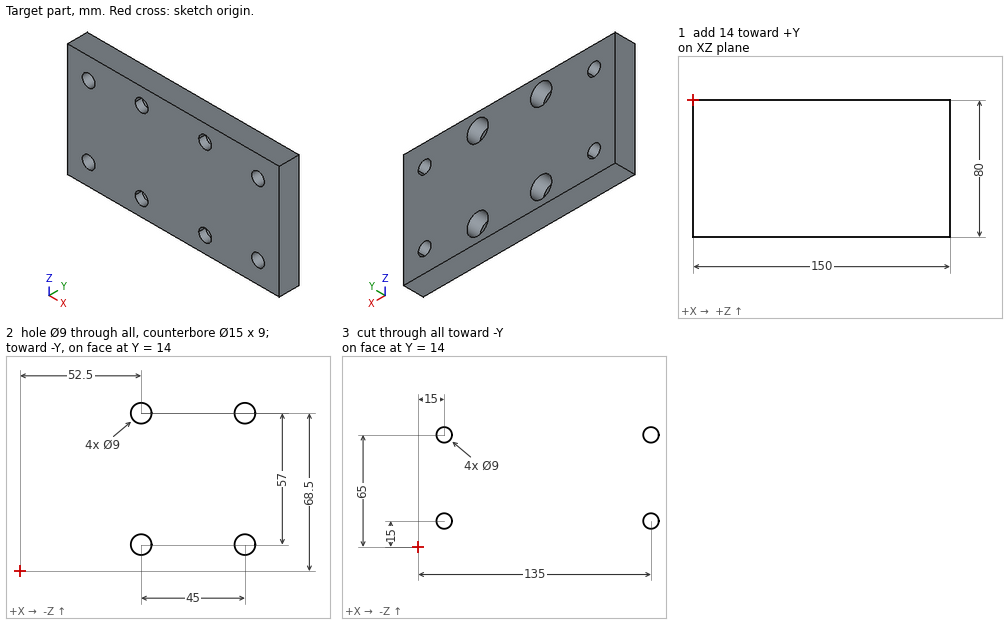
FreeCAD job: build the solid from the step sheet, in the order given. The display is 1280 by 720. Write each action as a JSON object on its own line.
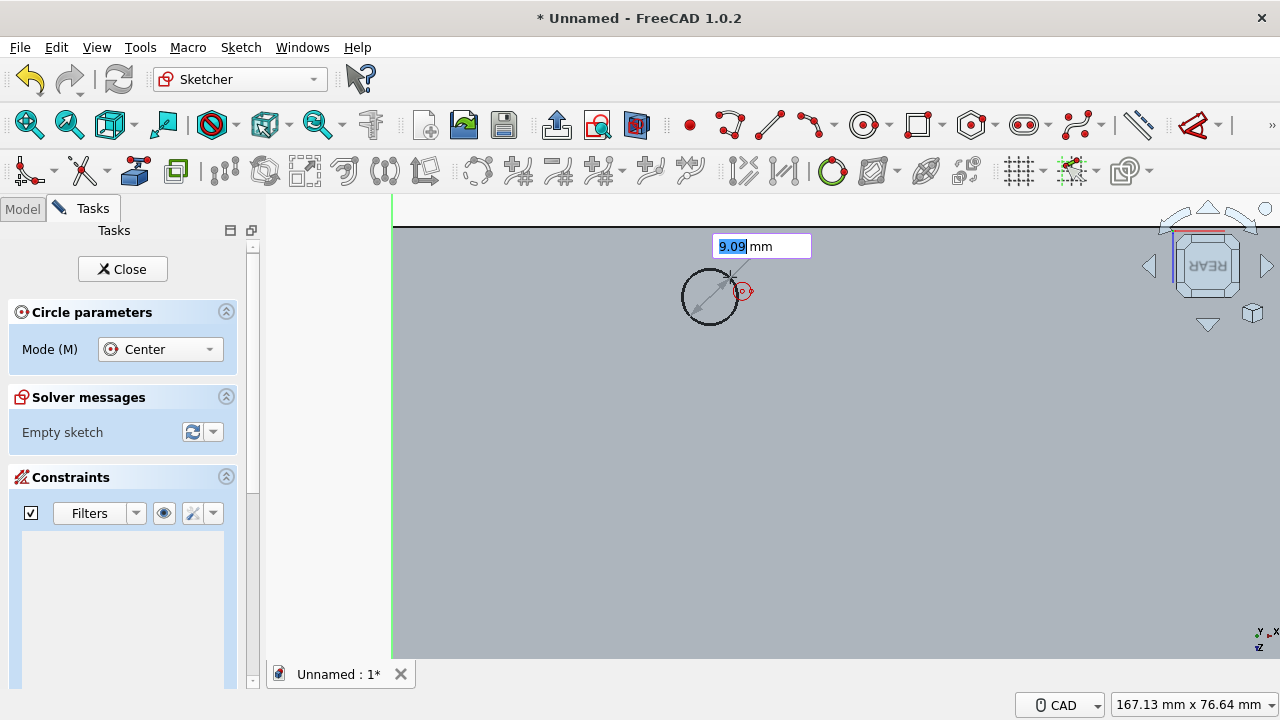
{"action": "type", "text": "9"}
{"action": "key", "text": "Return"}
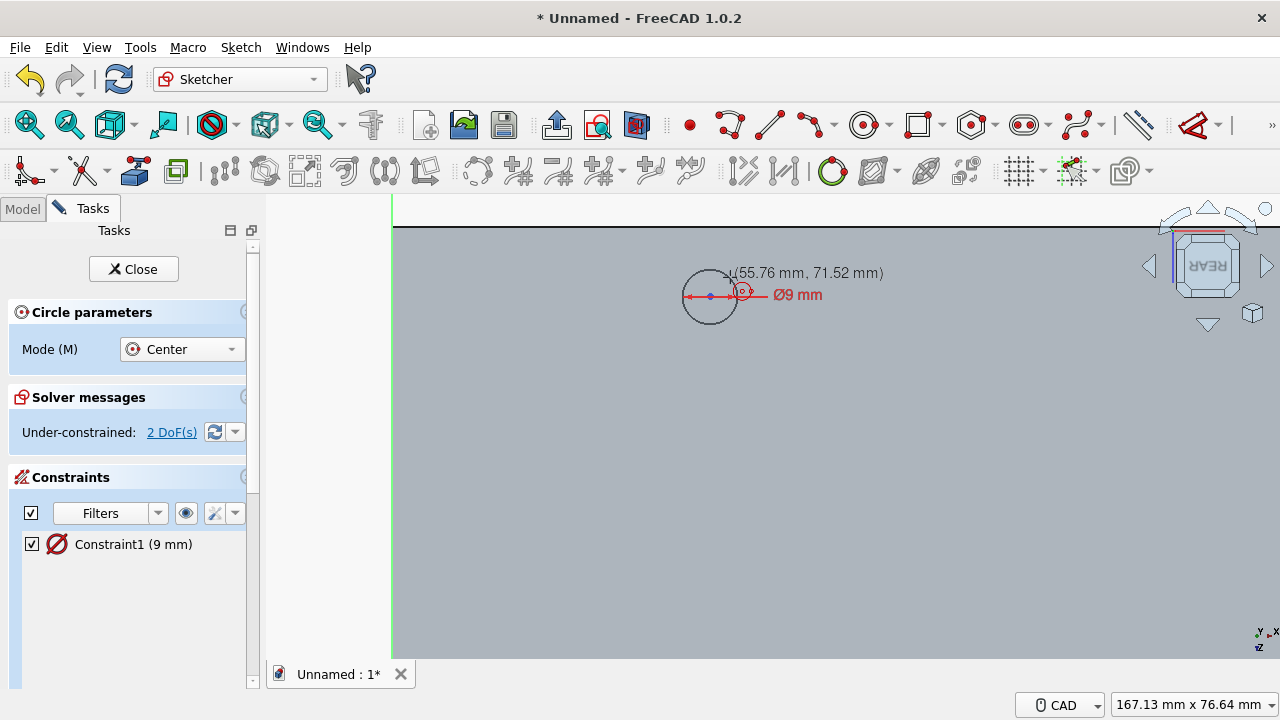
{"action": "scroll", "coordinate": [711, 296], "scroll_direction": "down", "scroll_amount": 2}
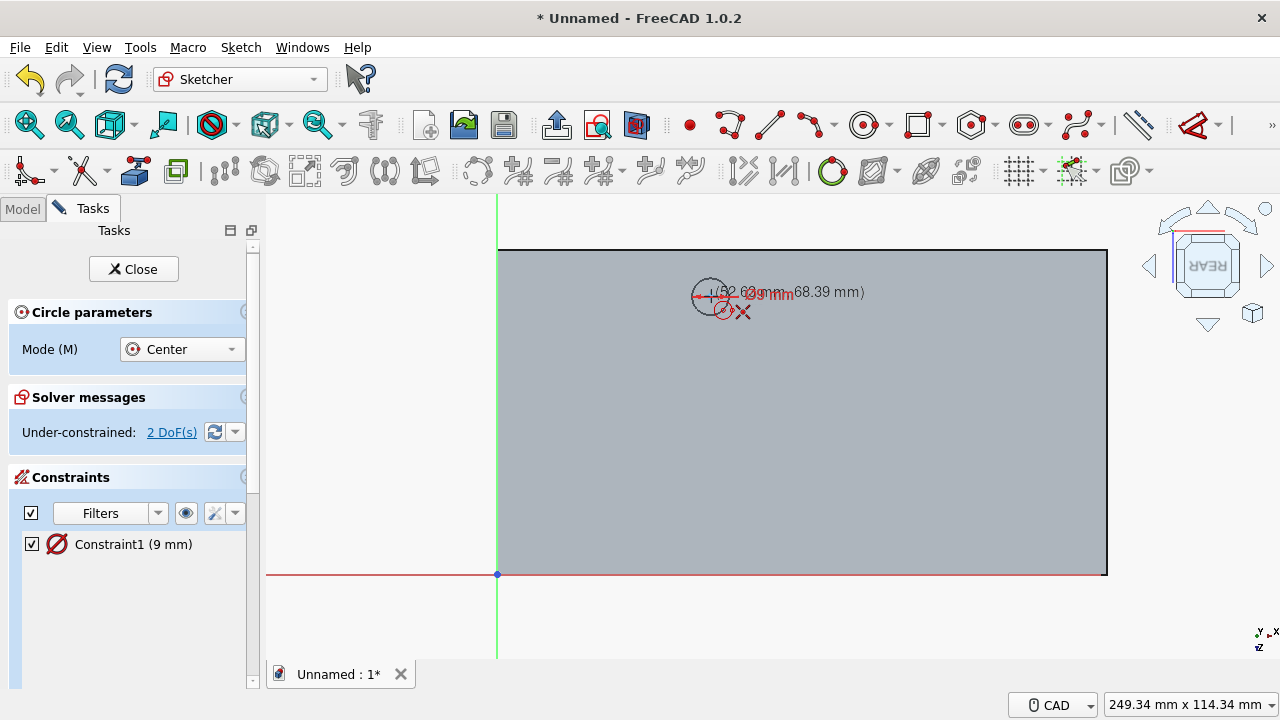
{"action": "scroll", "coordinate": [711, 528], "scroll_direction": "up", "scroll_amount": 2}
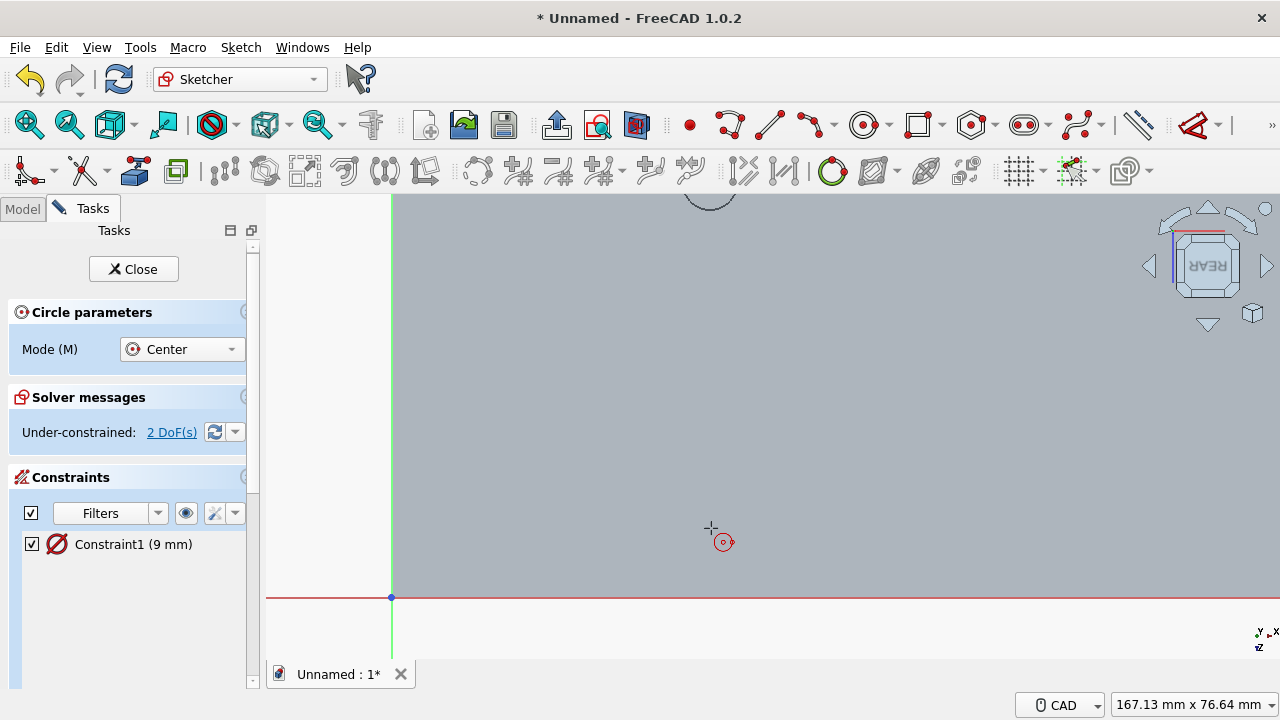
{"action": "left_click", "coordinate": [710, 528]}
{"action": "mouse_move", "coordinate": [730, 509]}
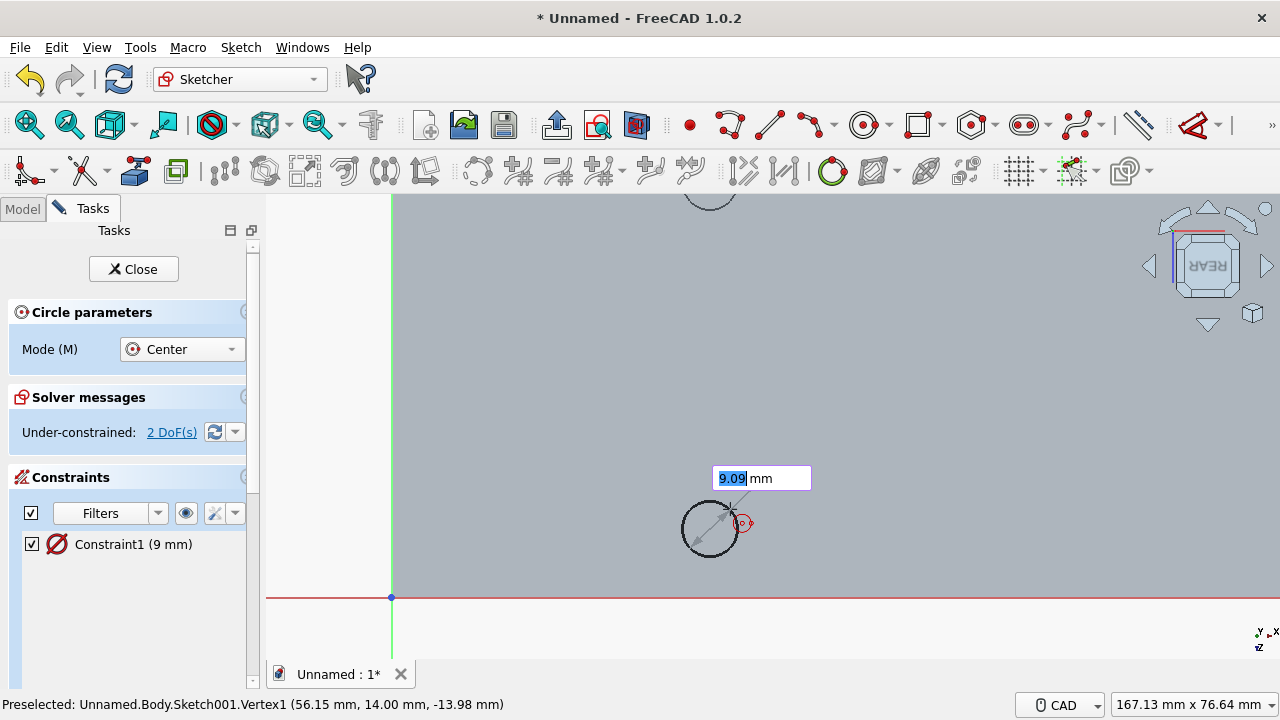
{"action": "type", "text": "9"}
{"action": "key", "text": "Return"}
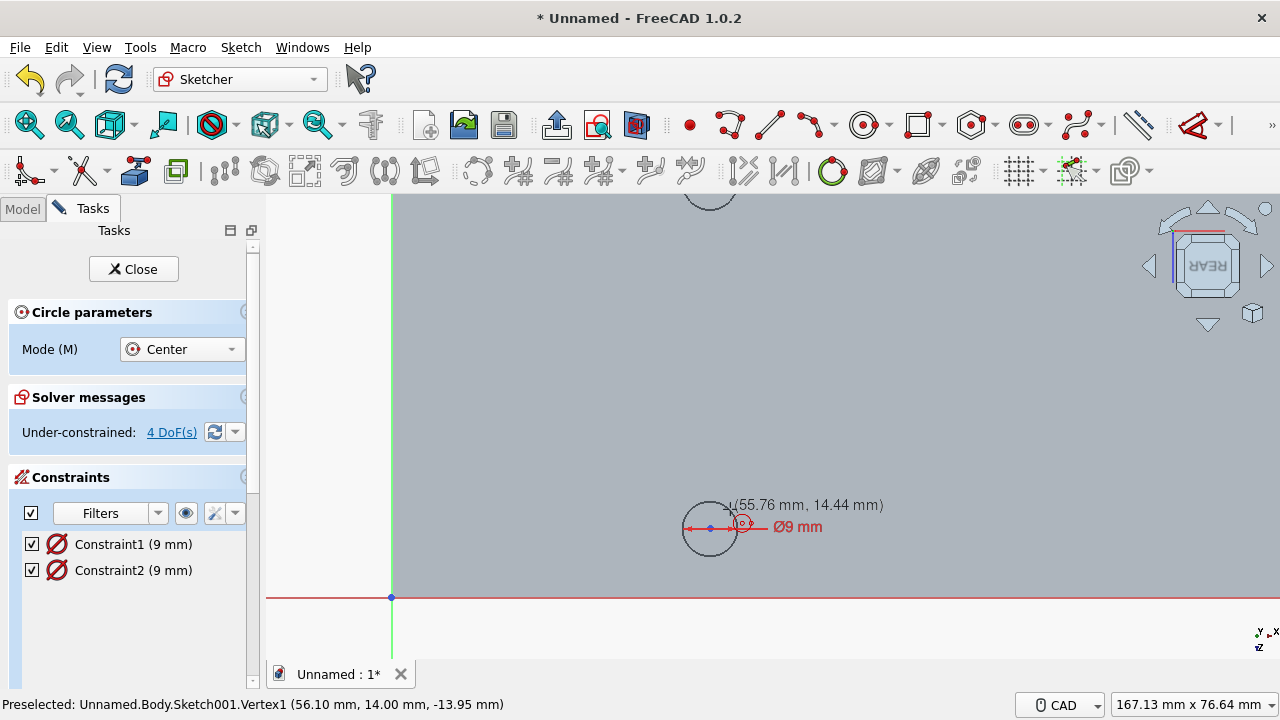
{"action": "left_click", "coordinate": [983, 528]}
{"action": "mouse_move", "coordinate": [1003, 509]}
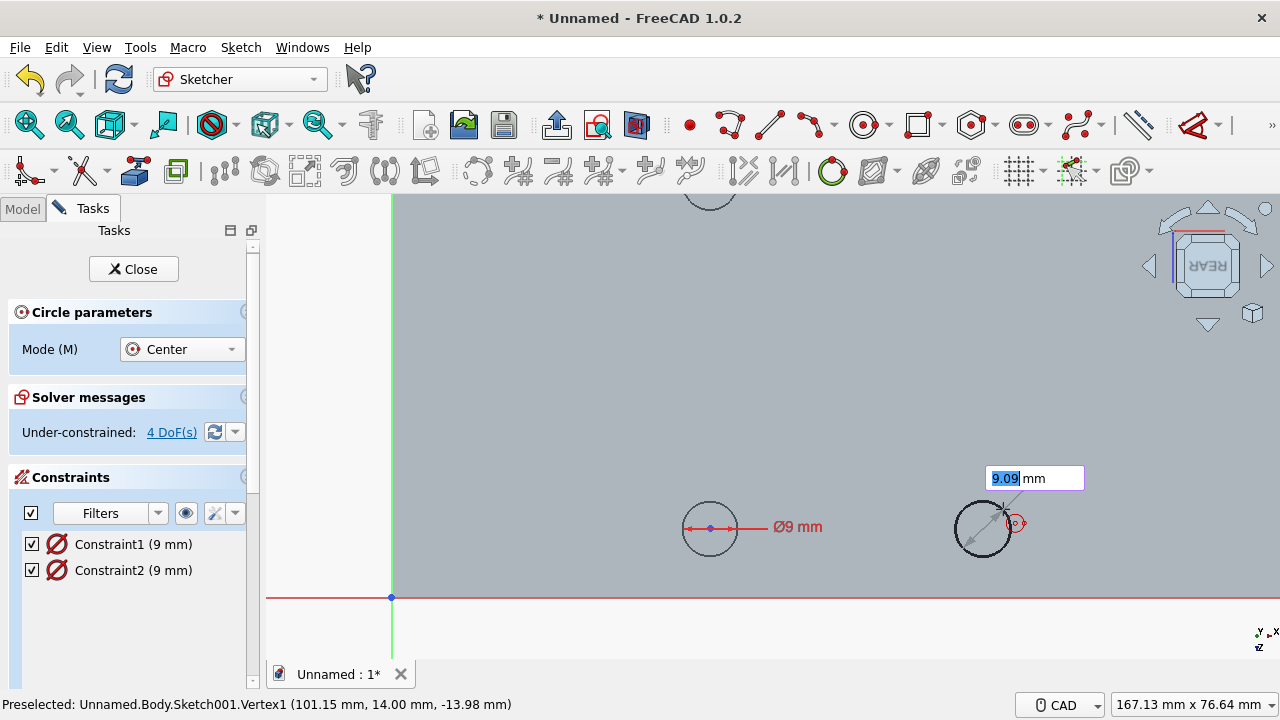
{"action": "type", "text": "9"}
{"action": "key", "text": "Return"}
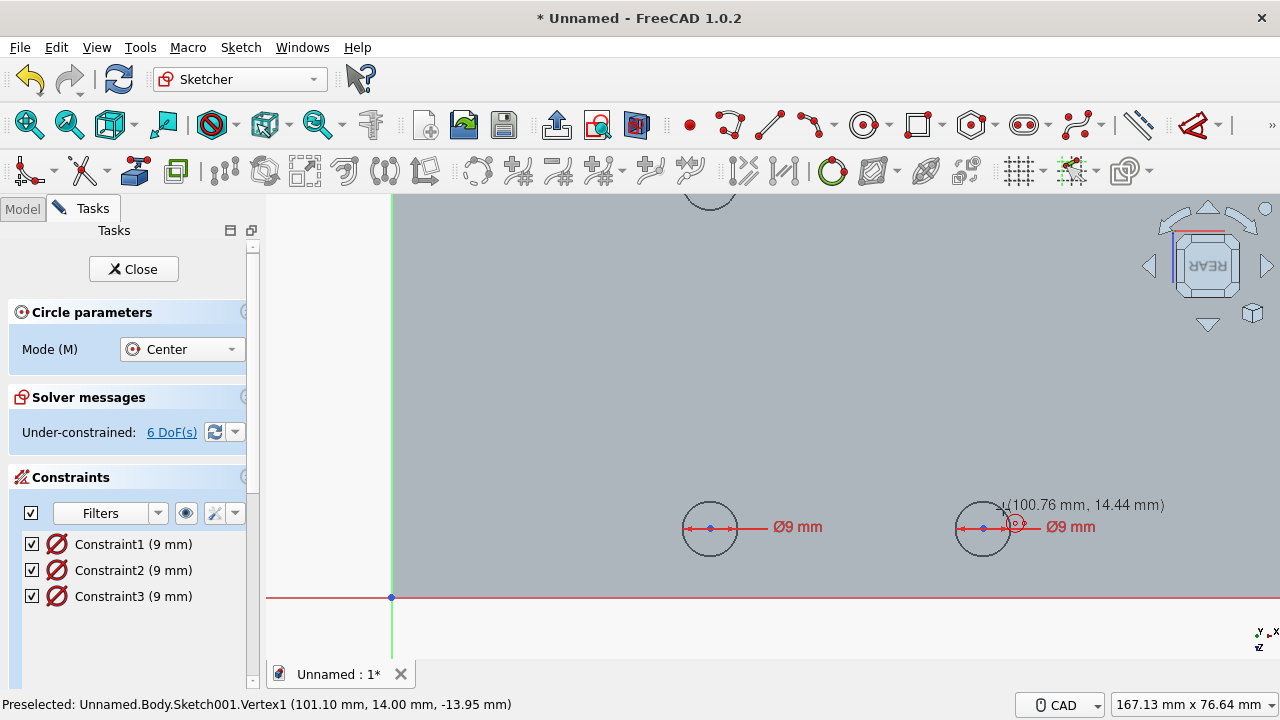
{"action": "scroll", "coordinate": [711, 529], "scroll_direction": "down", "scroll_amount": 2}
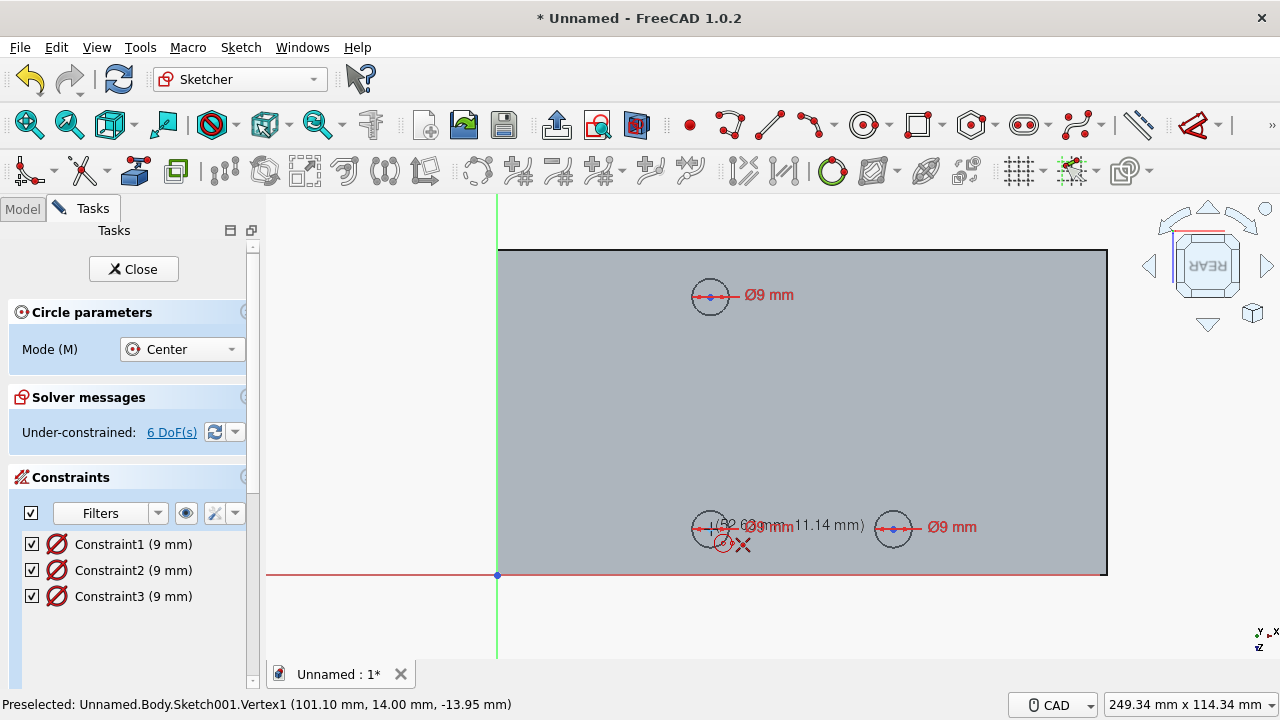
{"action": "scroll", "coordinate": [894, 297], "scroll_direction": "up", "scroll_amount": 2}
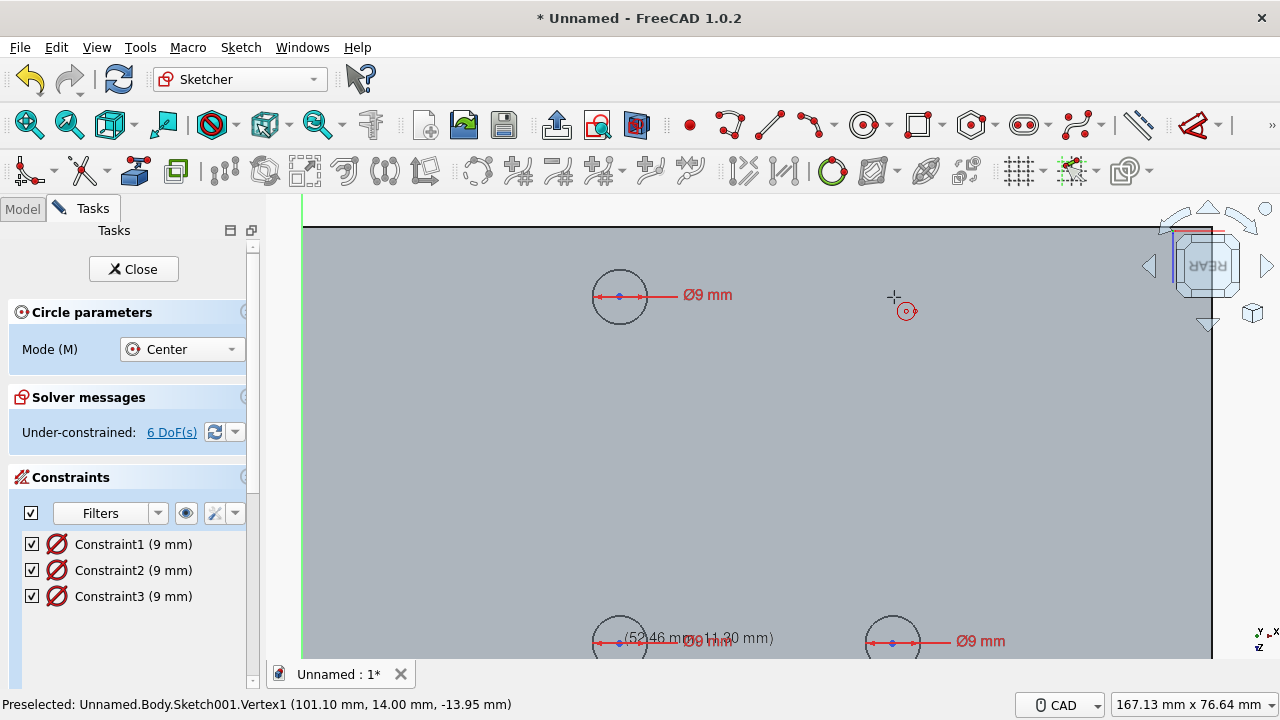
{"action": "left_click", "coordinate": [893, 296]}
{"action": "mouse_move", "coordinate": [912, 277]}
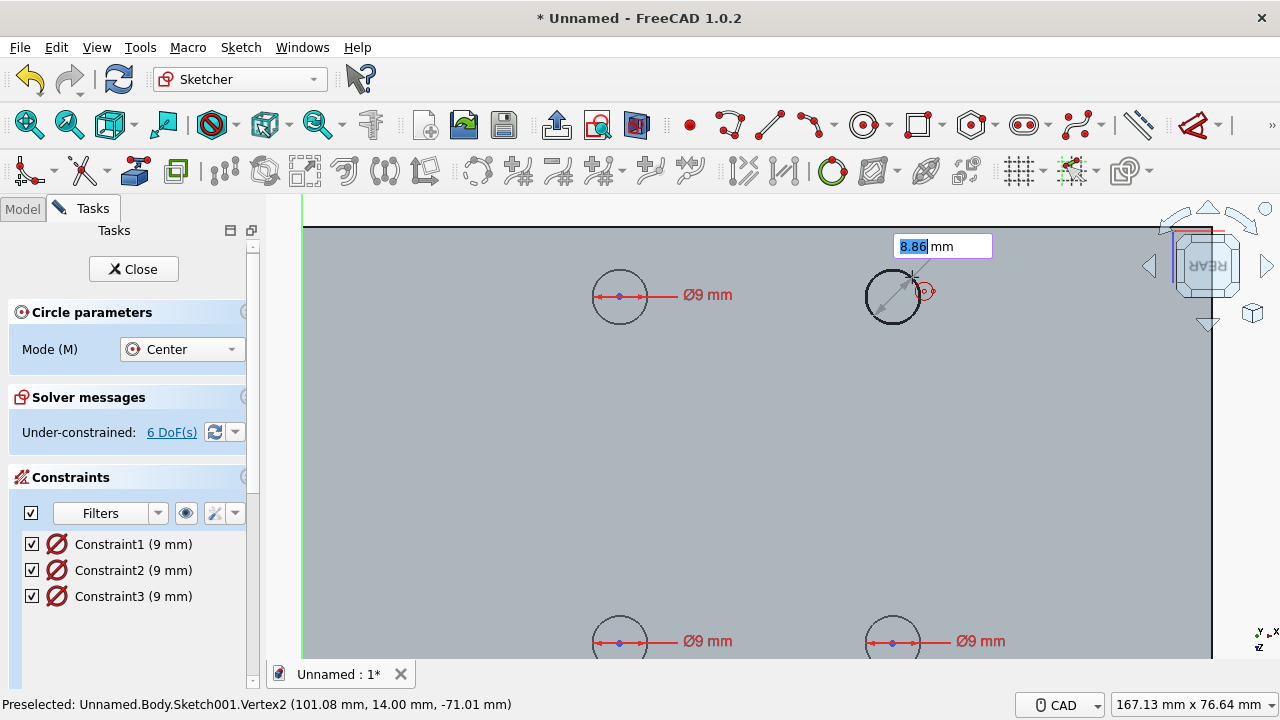
{"action": "type", "text": "9"}
{"action": "key", "text": "Return"}
{"action": "key", "text": "Escape"}